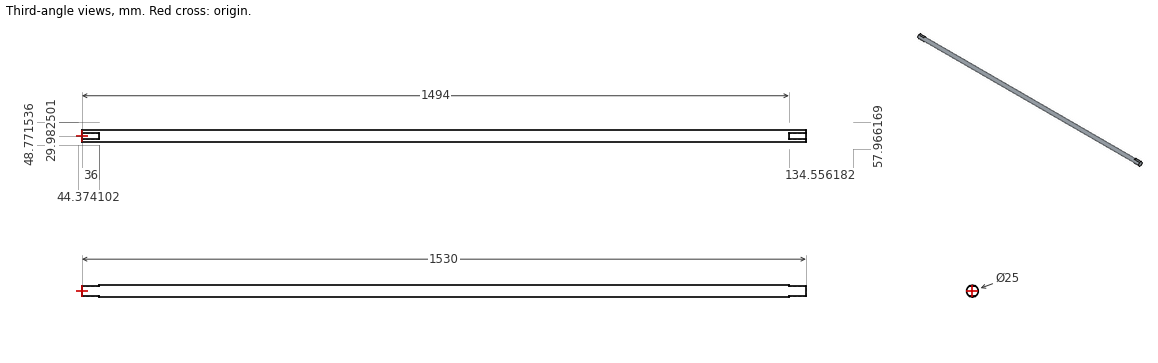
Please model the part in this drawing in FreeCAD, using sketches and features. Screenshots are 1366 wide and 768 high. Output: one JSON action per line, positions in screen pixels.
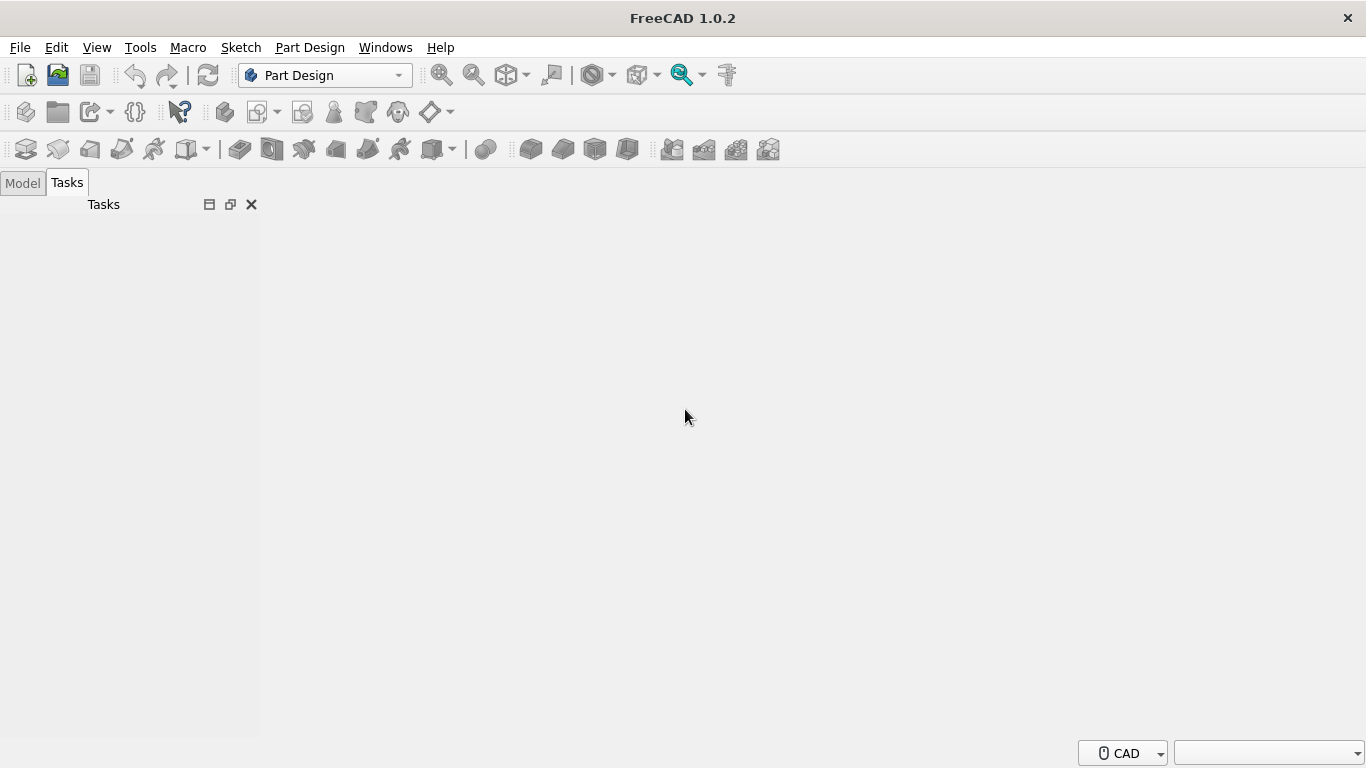
{"action": "left_click", "coordinate": [26, 76]}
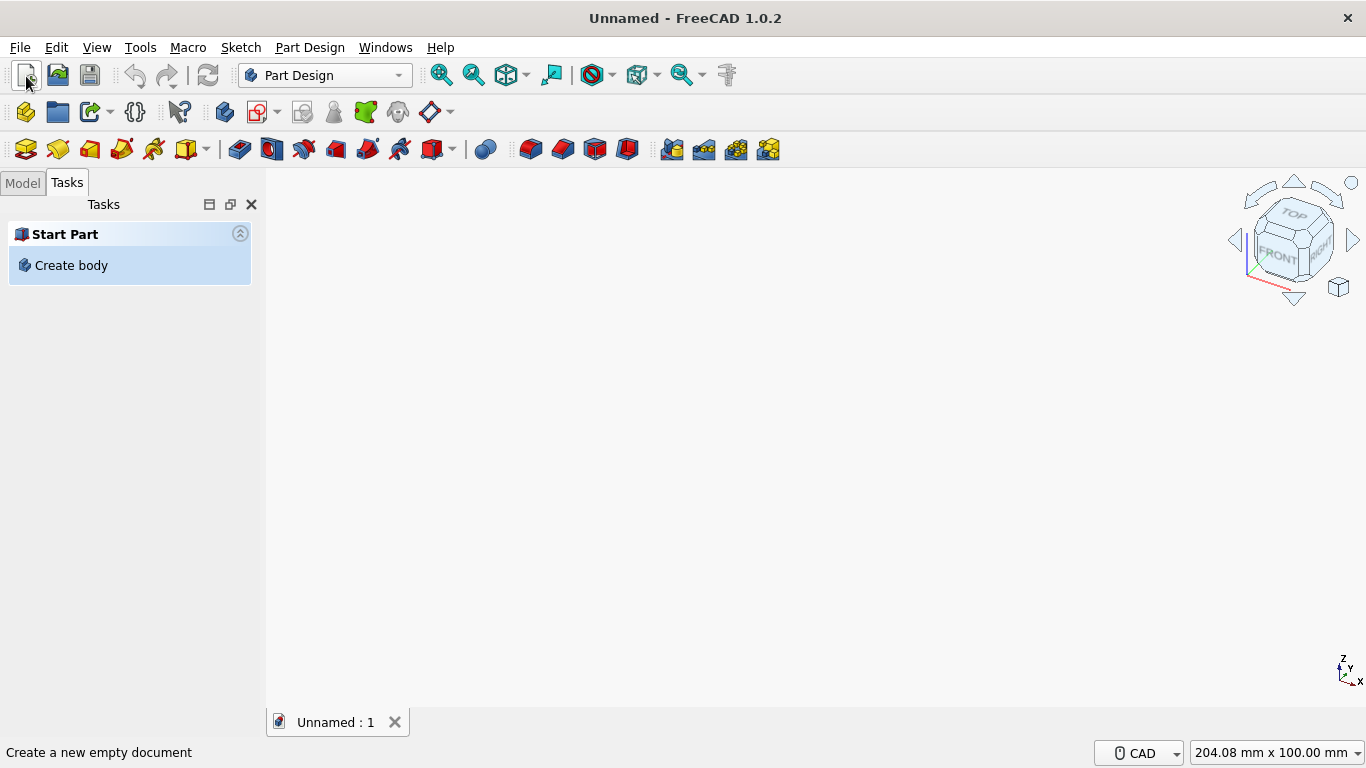
{"action": "left_click", "coordinate": [258, 112]}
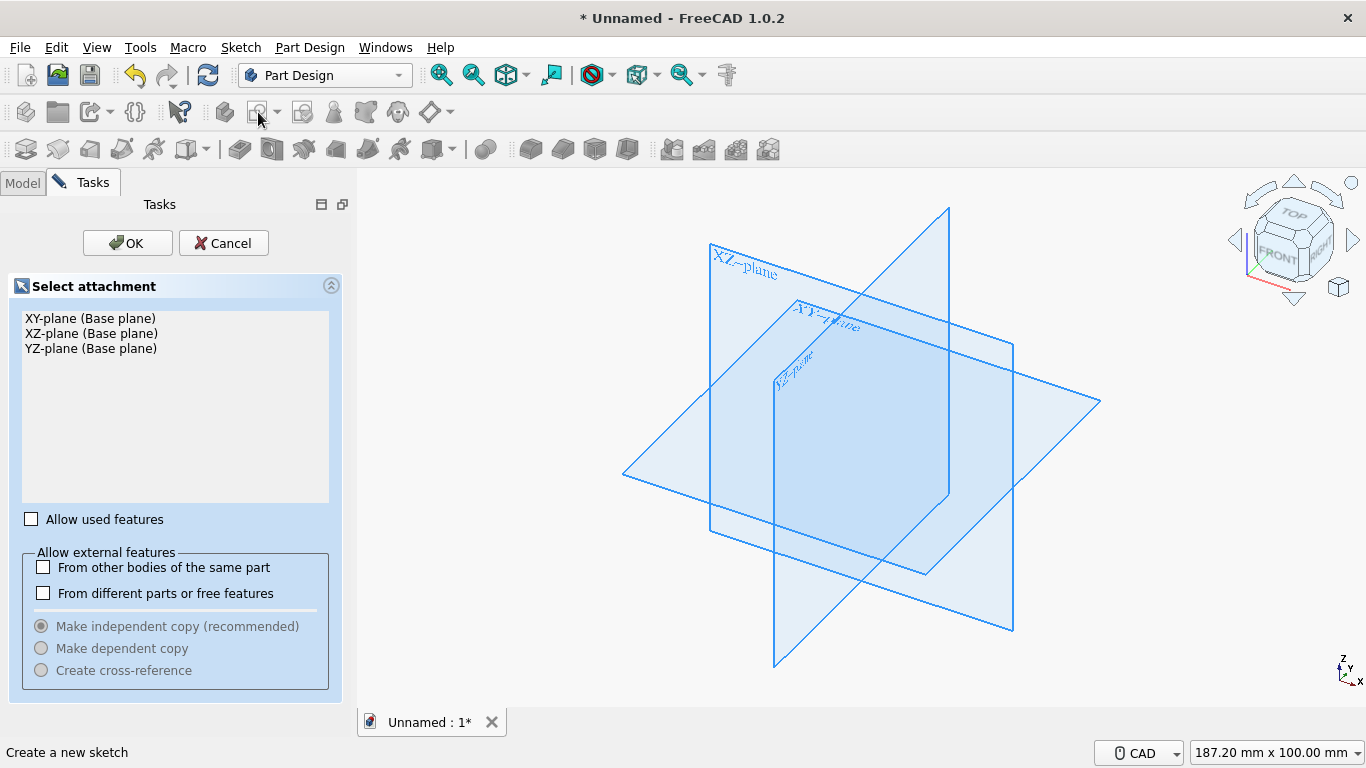
{"action": "left_click", "coordinate": [82, 348]}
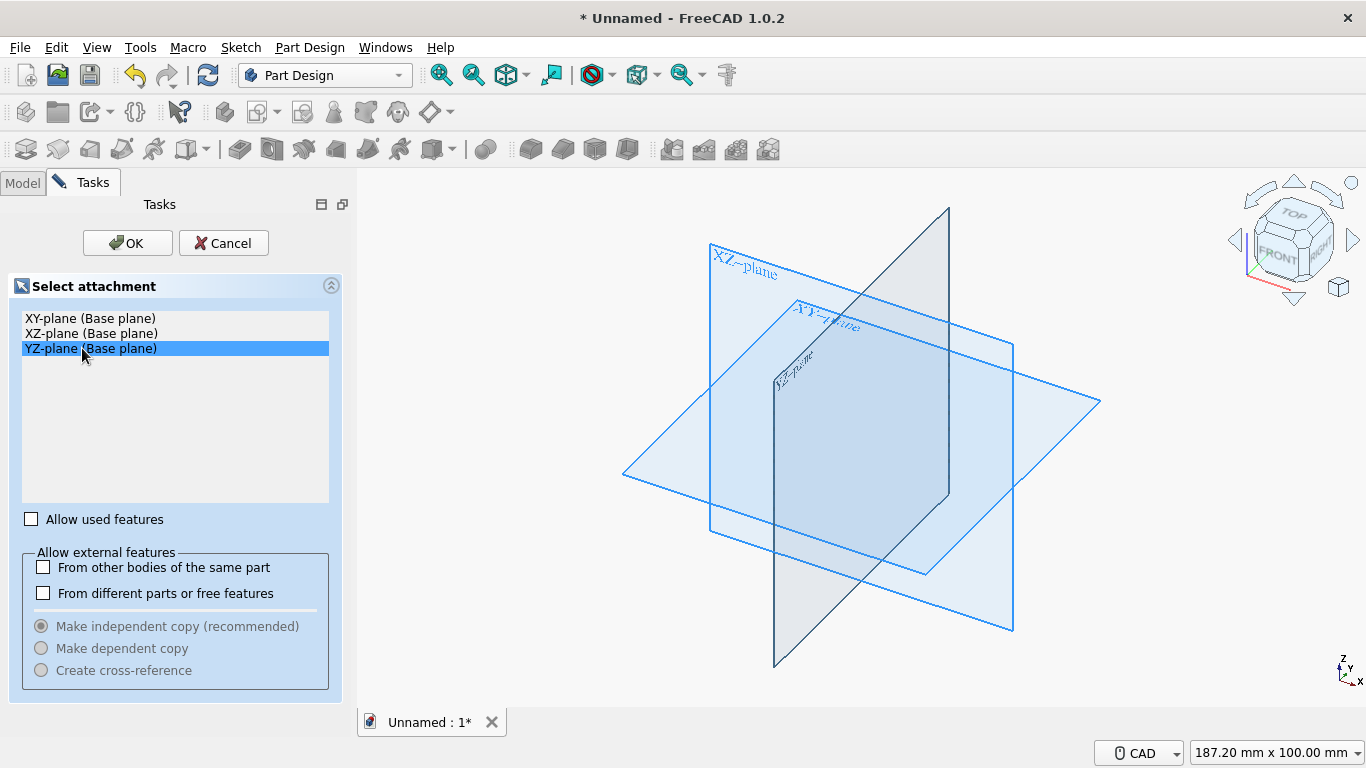
{"action": "left_click", "coordinate": [128, 243]}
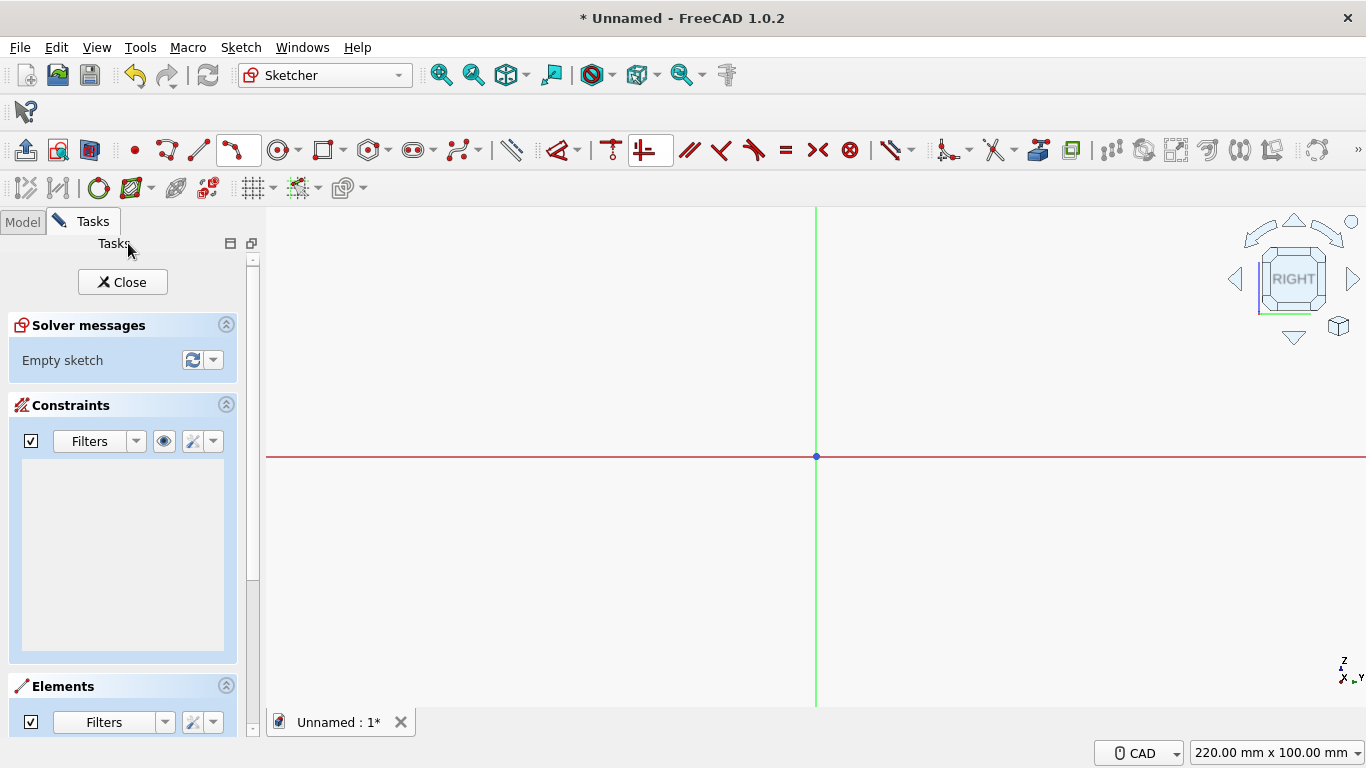
{"action": "scroll", "coordinate": [856, 457], "scroll_direction": "up", "scroll_amount": 5}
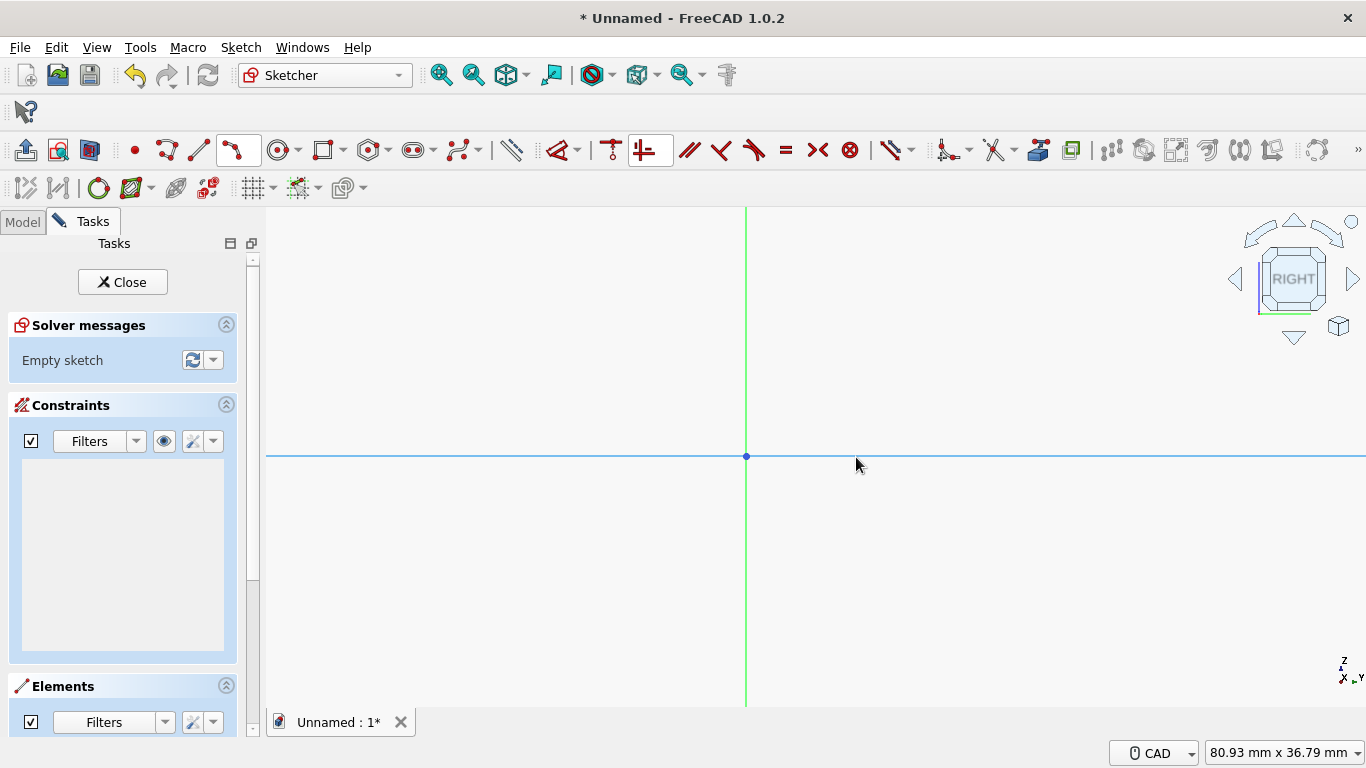
{"action": "left_click", "coordinate": [278, 150]}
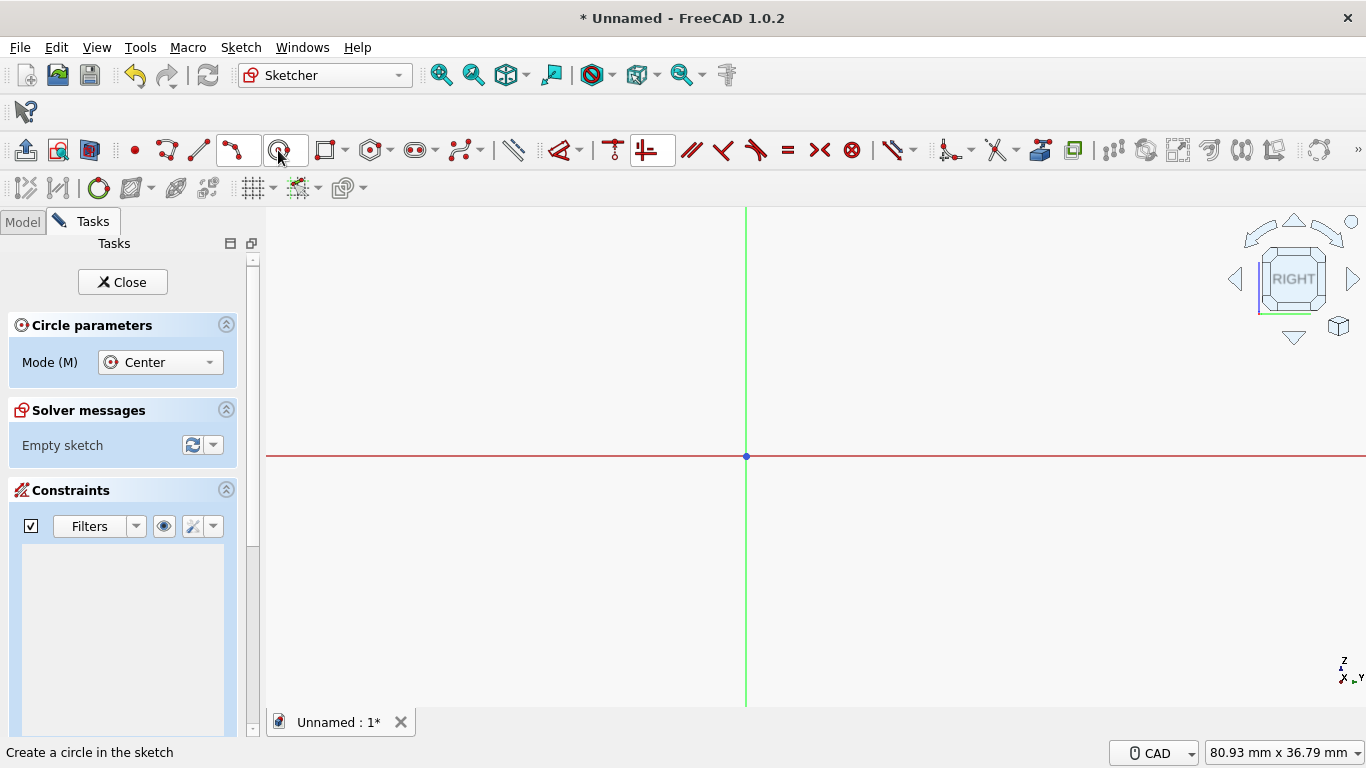
{"action": "left_click", "coordinate": [746, 456]}
{"action": "mouse_move", "coordinate": [866, 336]}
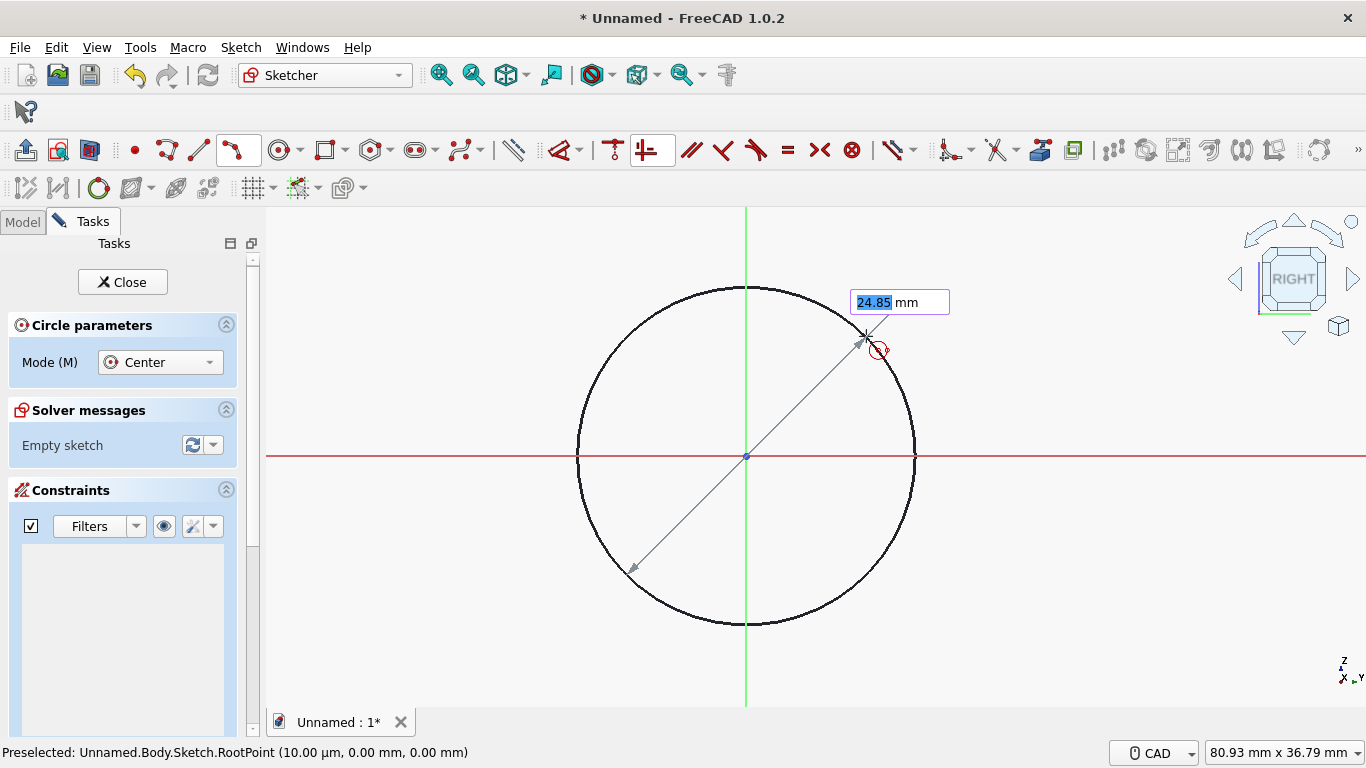
{"action": "type", "text": "25"}
{"action": "key", "text": "Return"}
{"action": "key", "text": "Escape"}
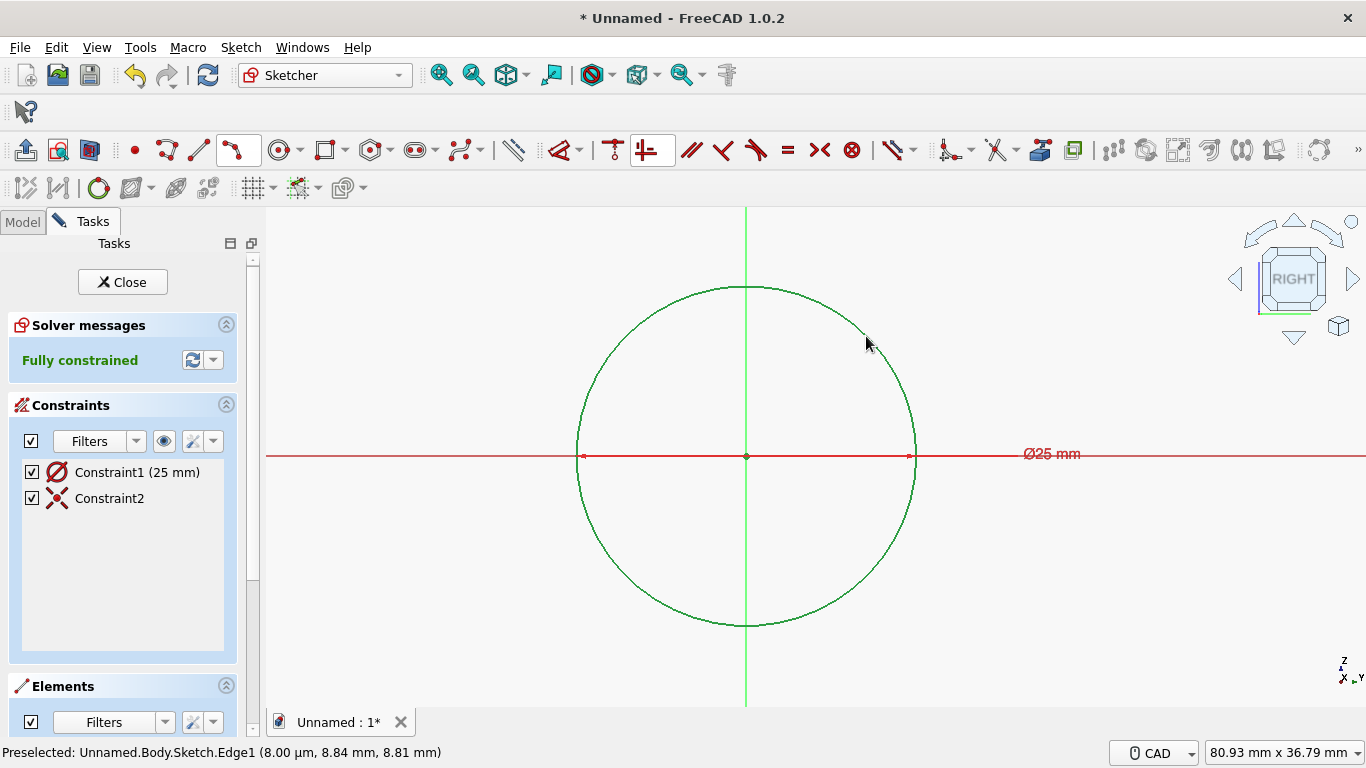
{"action": "left_click", "coordinate": [123, 282]}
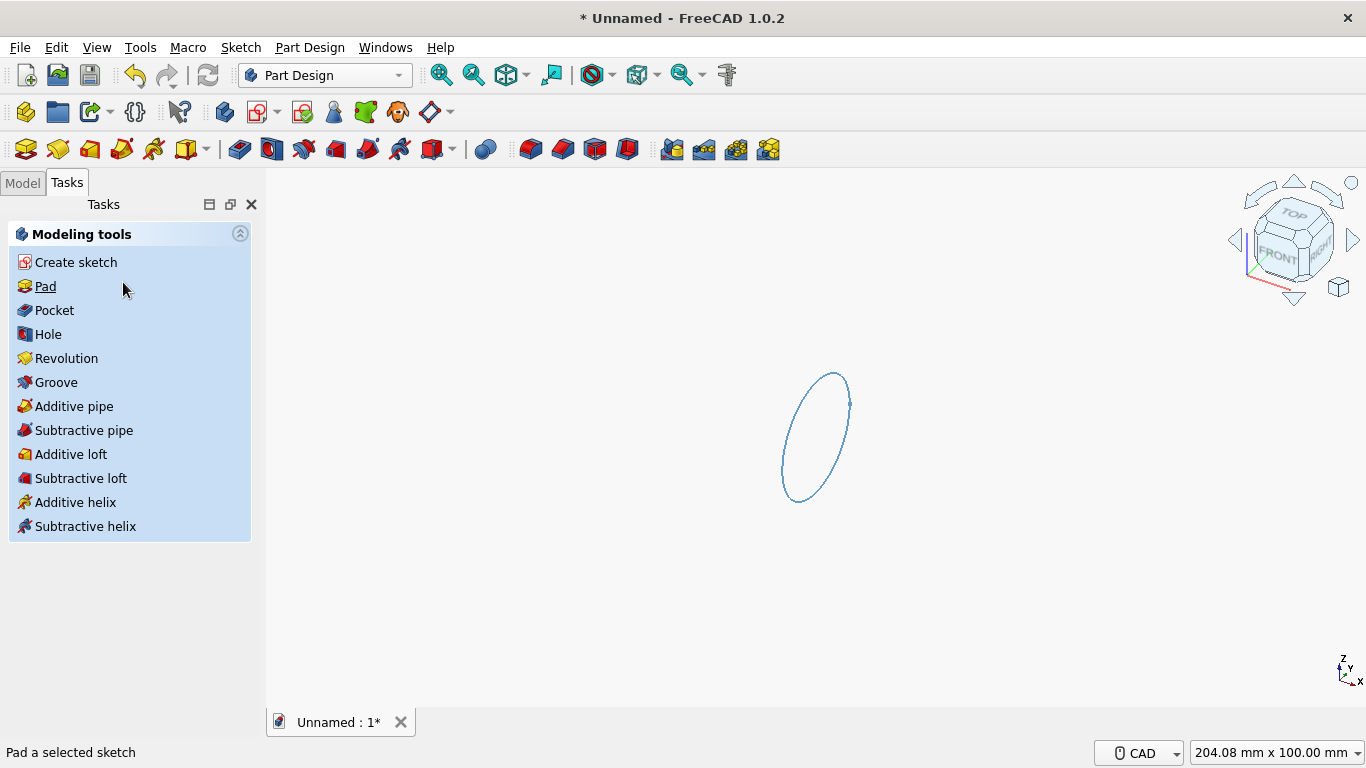
{"action": "left_click", "coordinate": [26, 150]}